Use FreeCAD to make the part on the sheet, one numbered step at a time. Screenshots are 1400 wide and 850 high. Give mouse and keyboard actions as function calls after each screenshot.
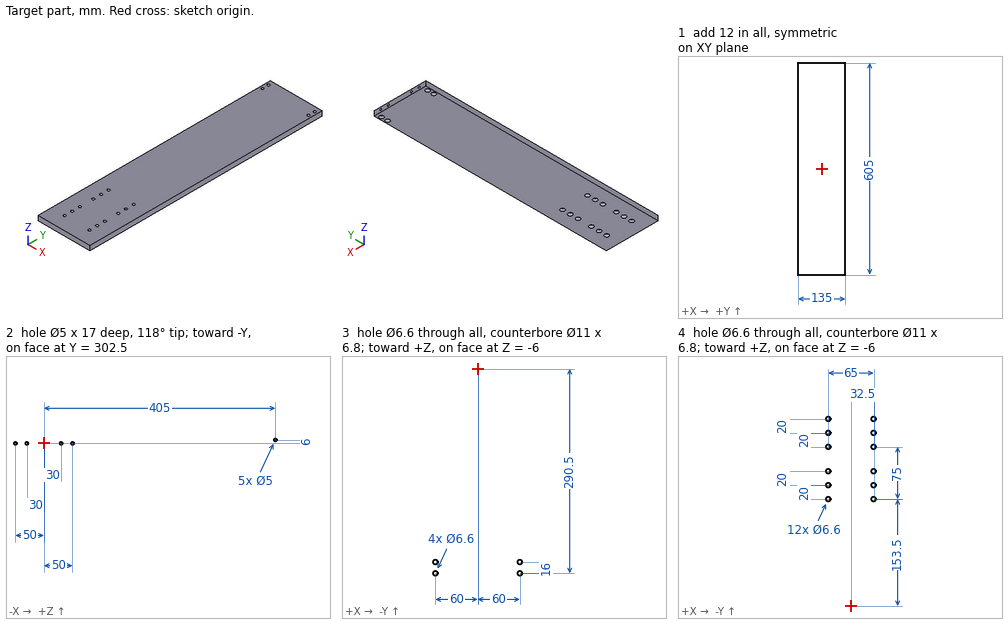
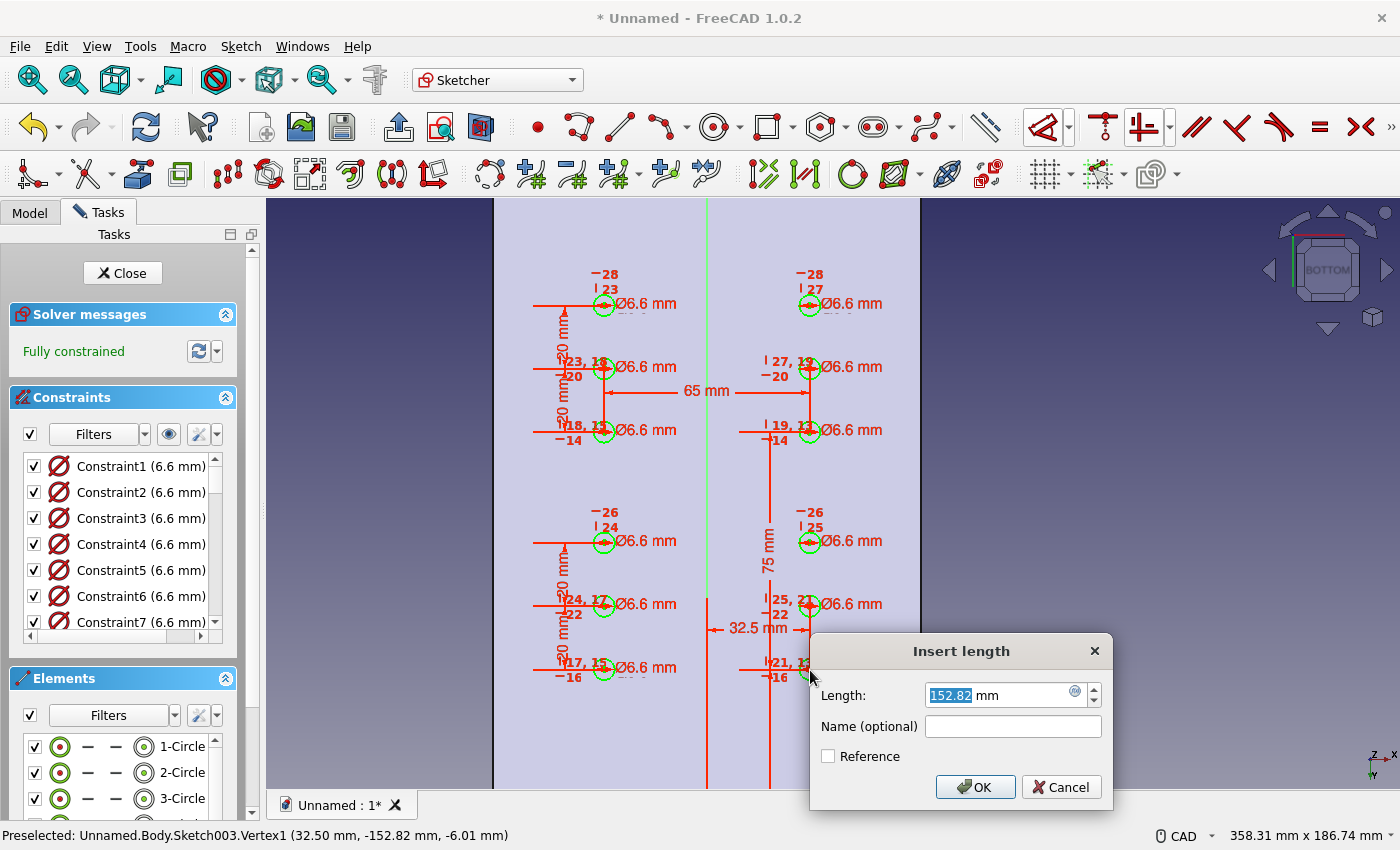
text(153.5)
key(Return)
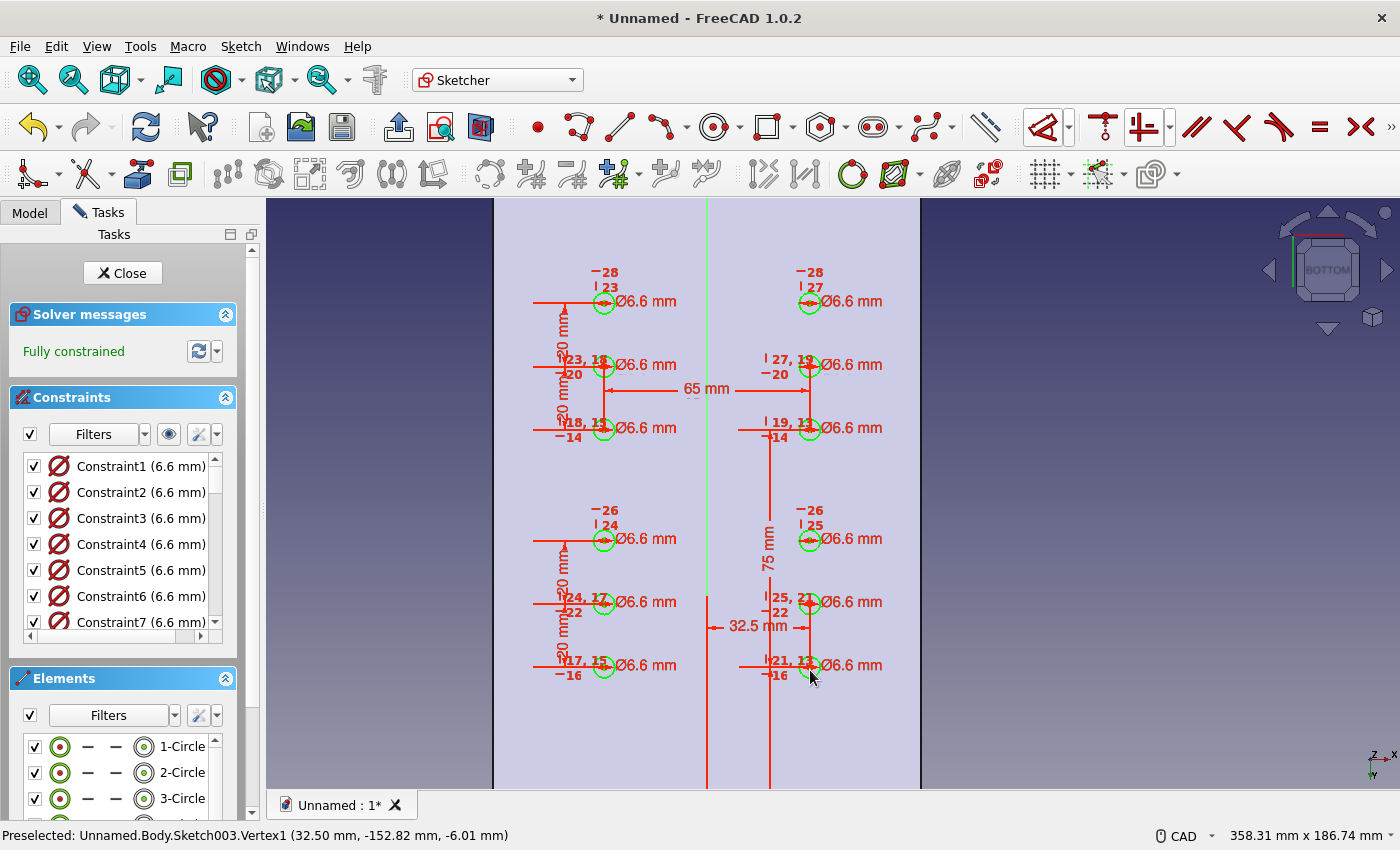
click(123, 273)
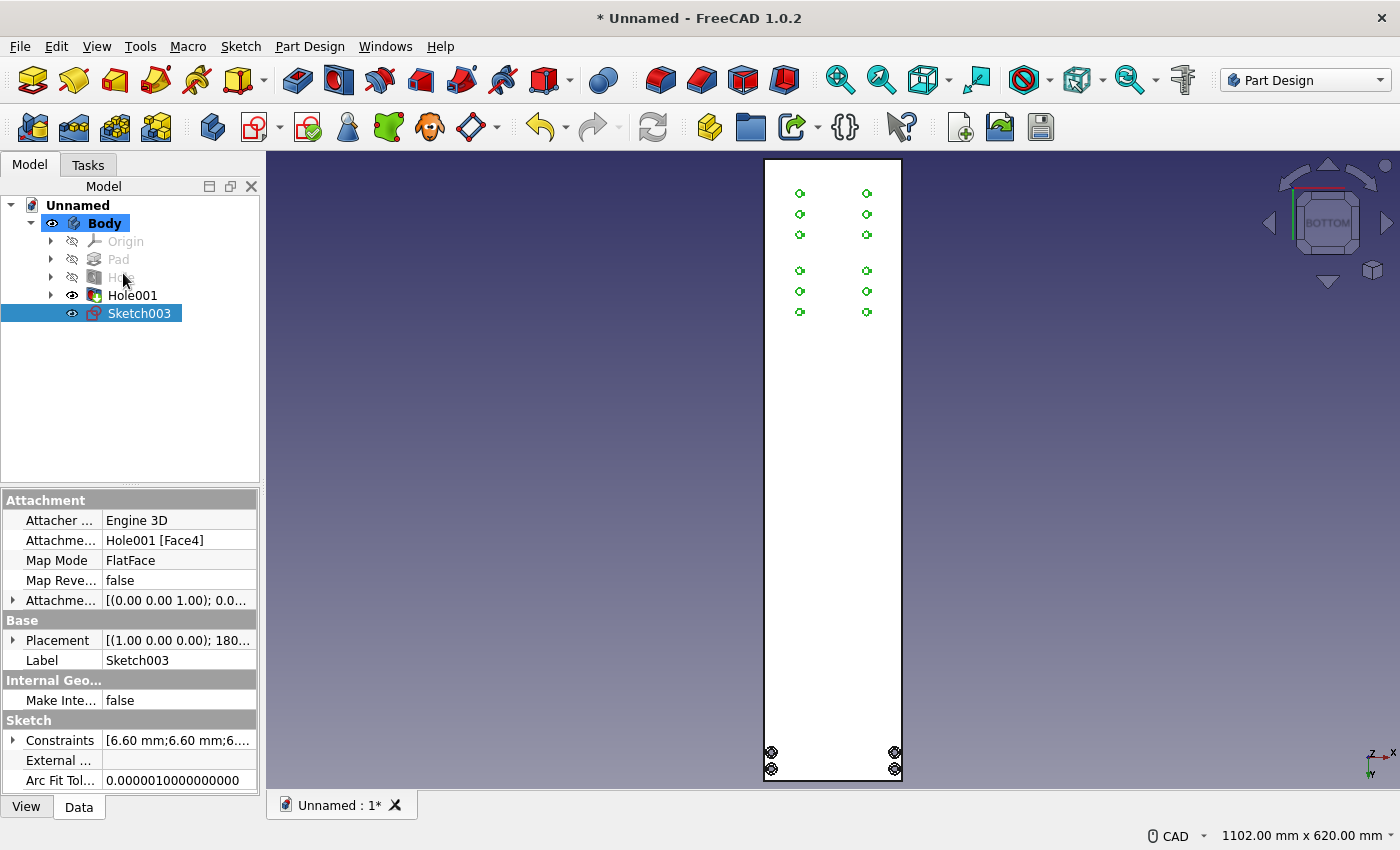
click(339, 80)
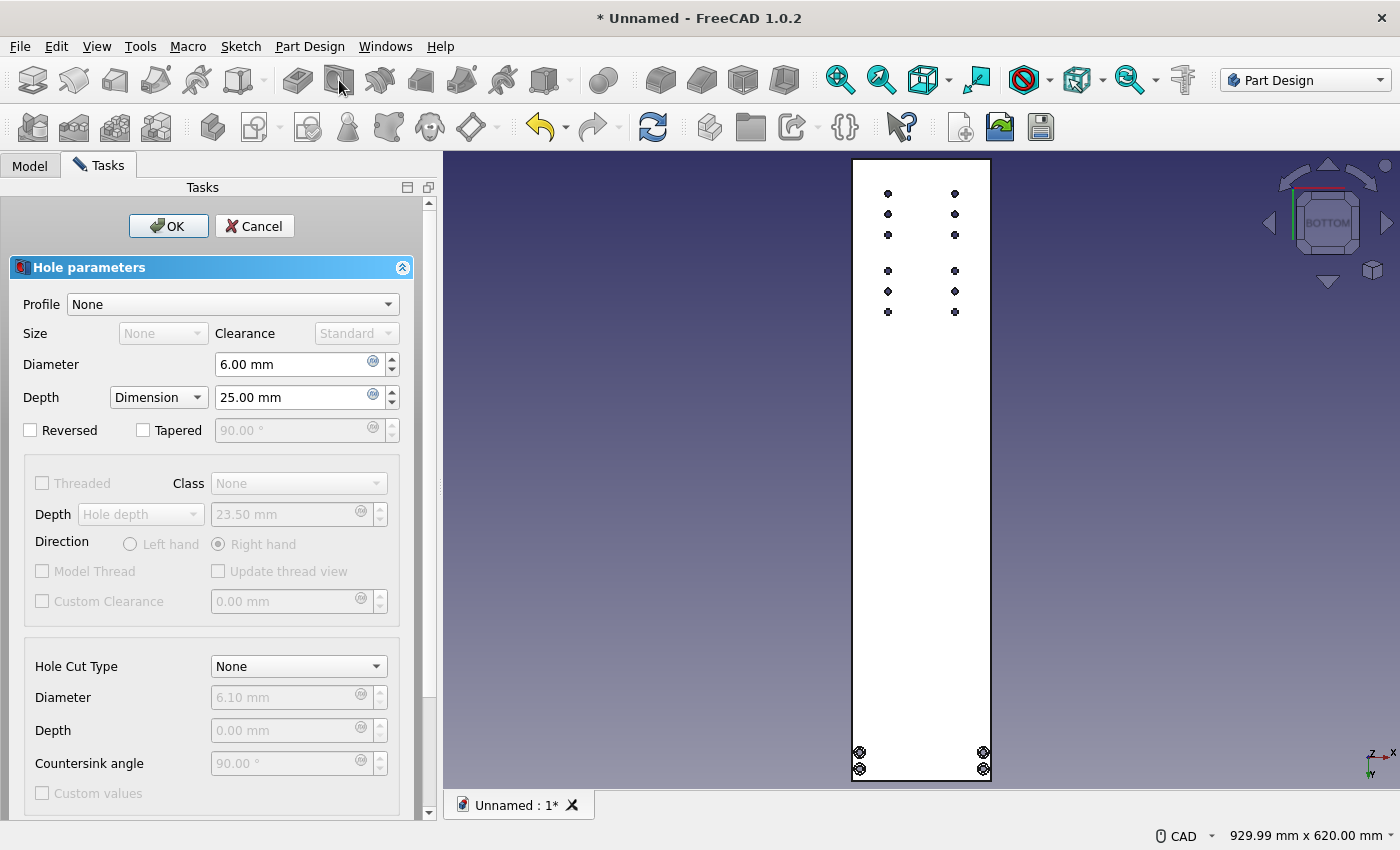
triple_click(300, 364)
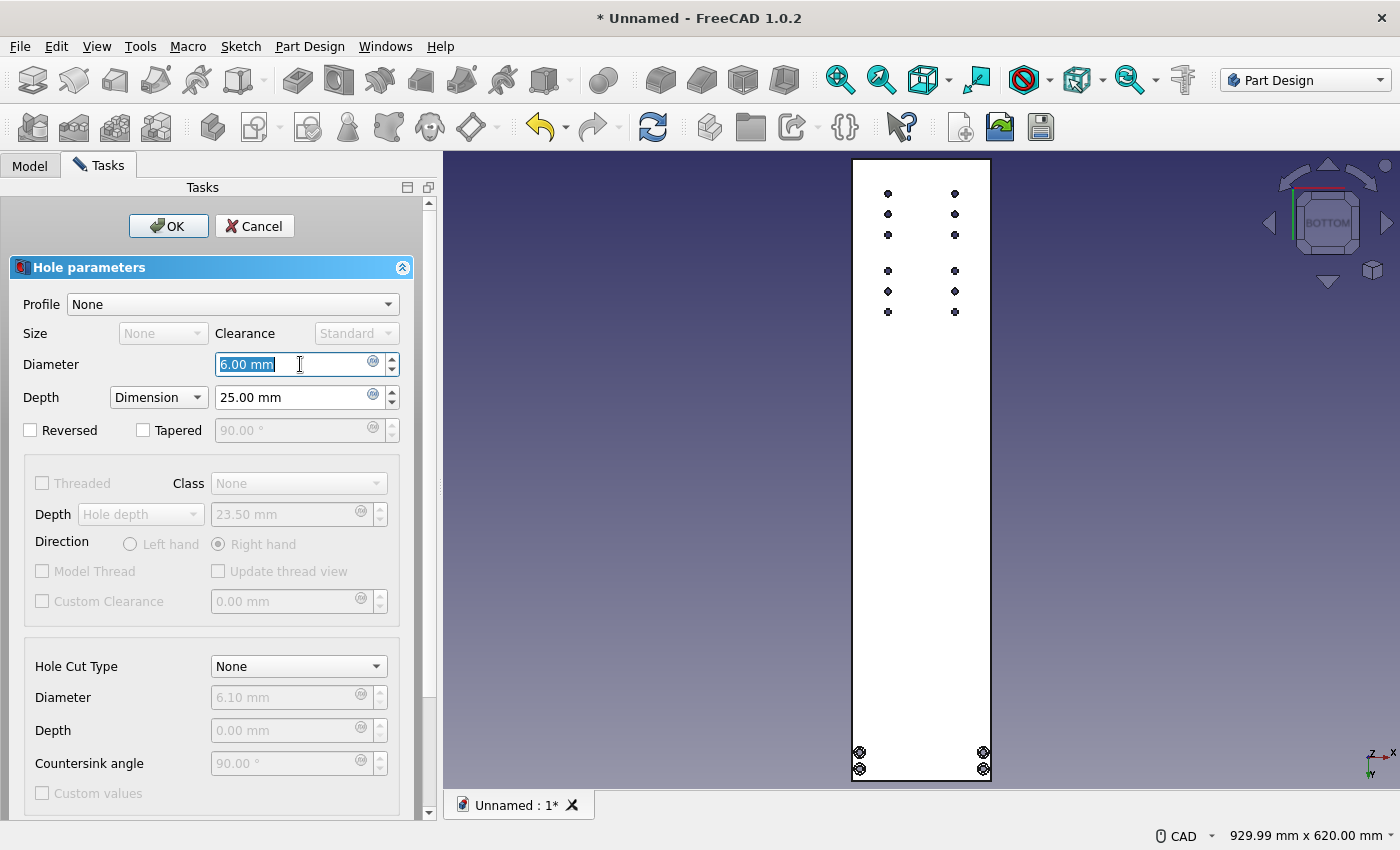
text(6.6)
key(Tab)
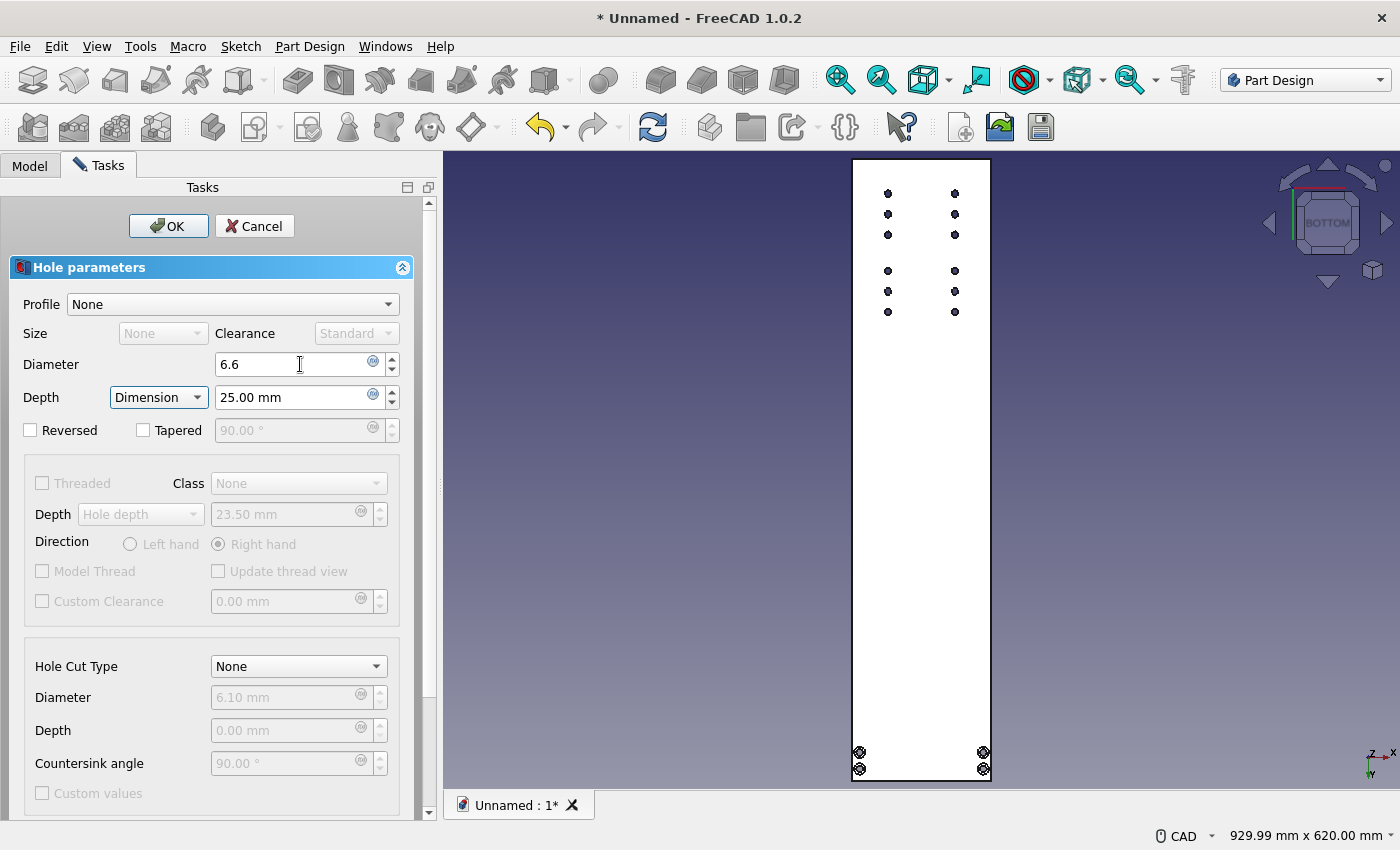
click(160, 398)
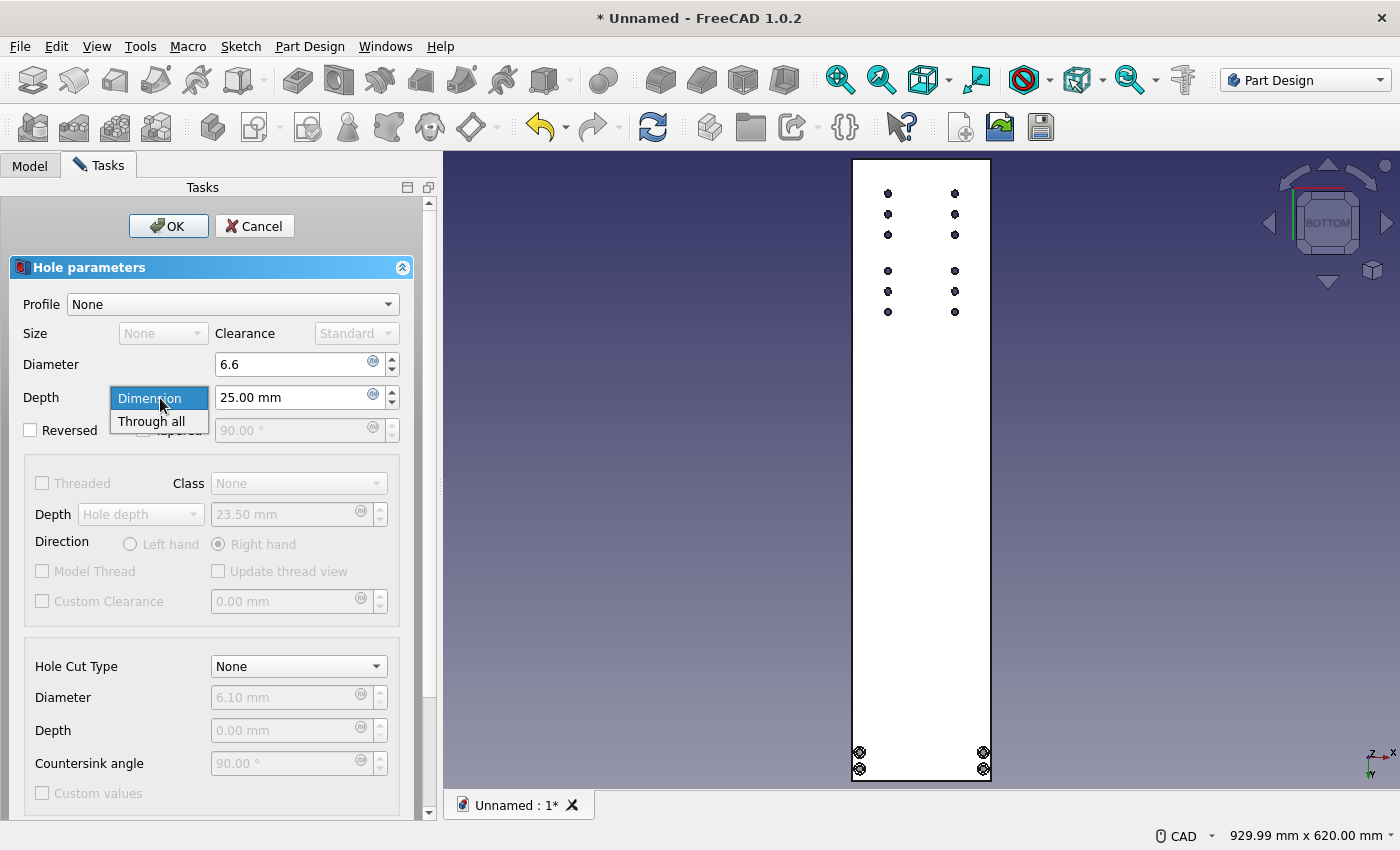
click(158, 422)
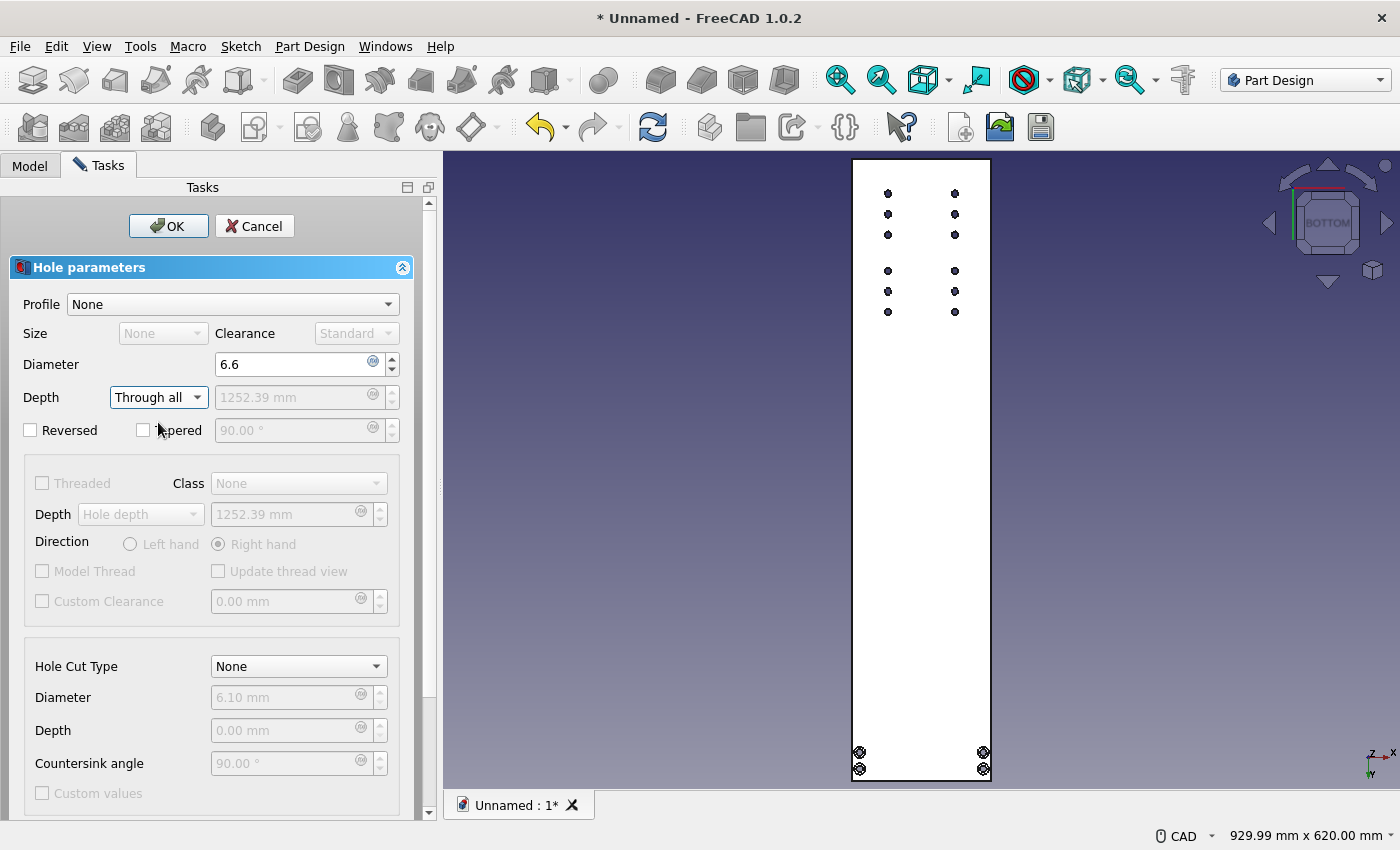
click(300, 666)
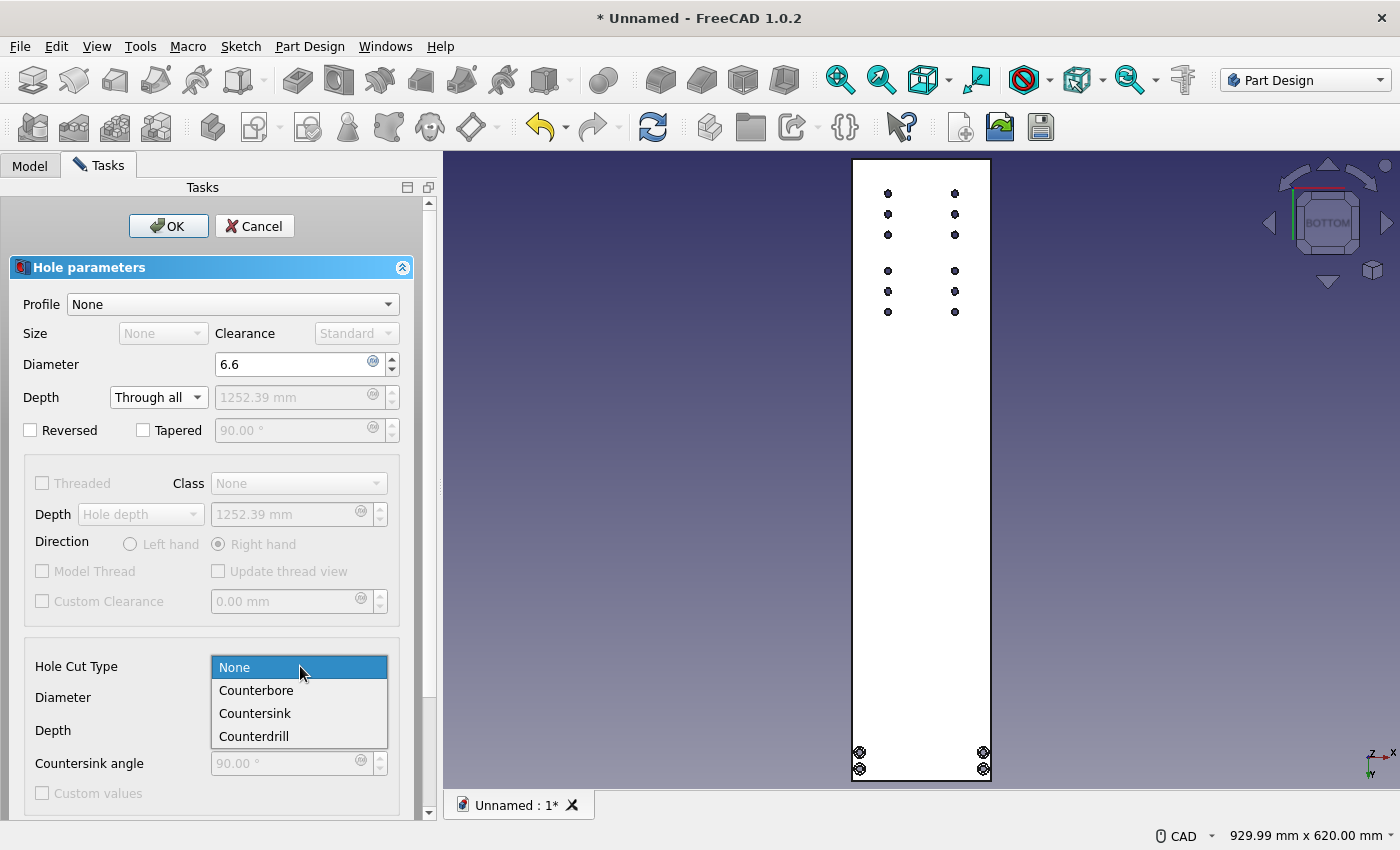
click(298, 690)